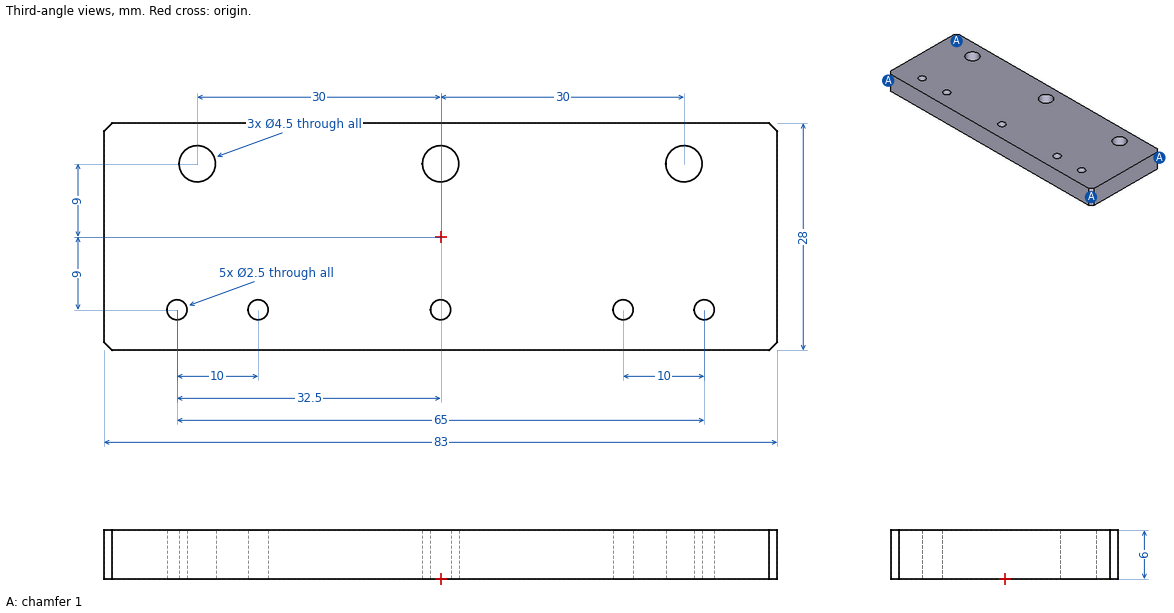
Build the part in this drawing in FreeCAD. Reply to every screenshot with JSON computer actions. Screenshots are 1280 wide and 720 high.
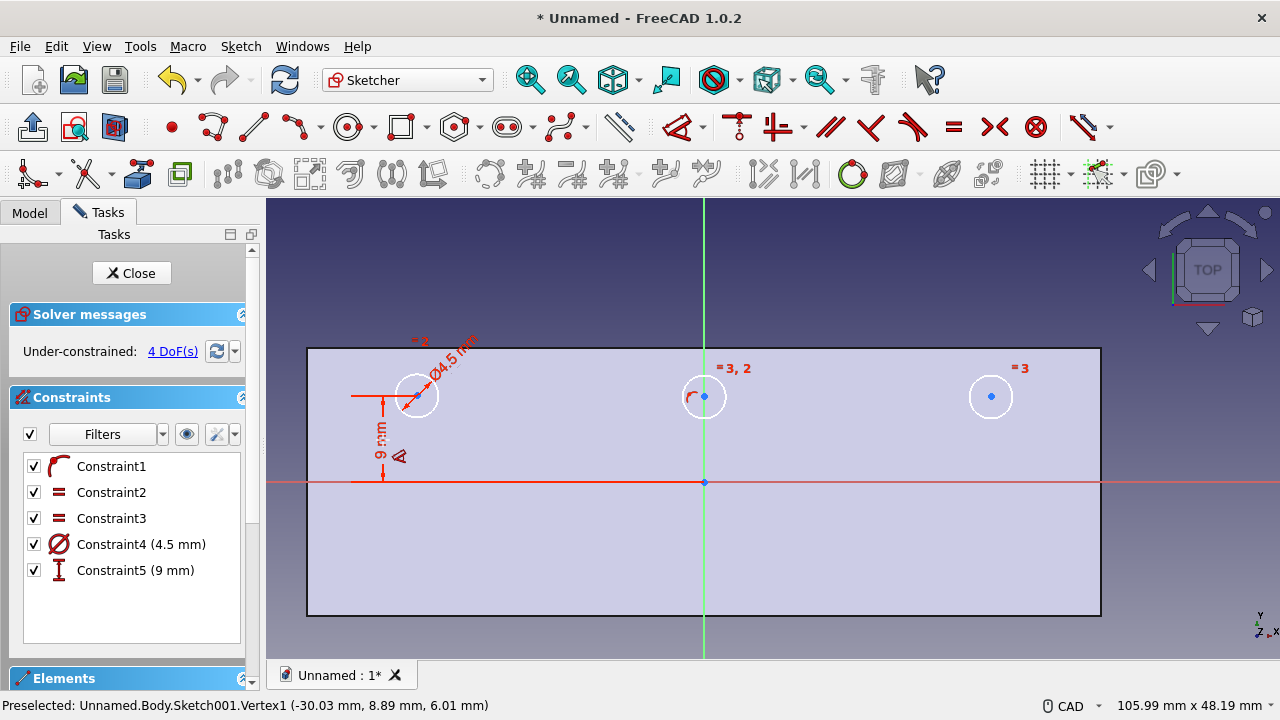
{"action": "left_click", "coordinate": [704, 397]}
{"action": "left_click", "coordinate": [738, 440]}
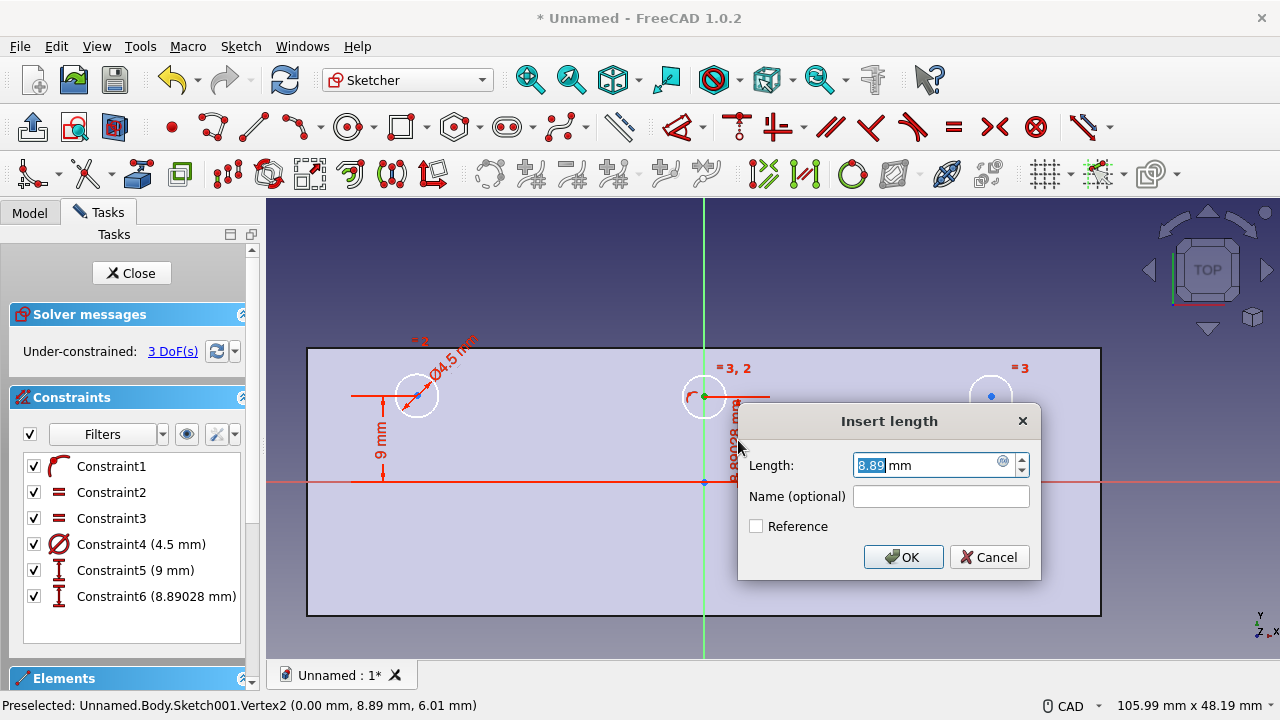
{"action": "type", "text": "9"}
{"action": "key", "text": "Return"}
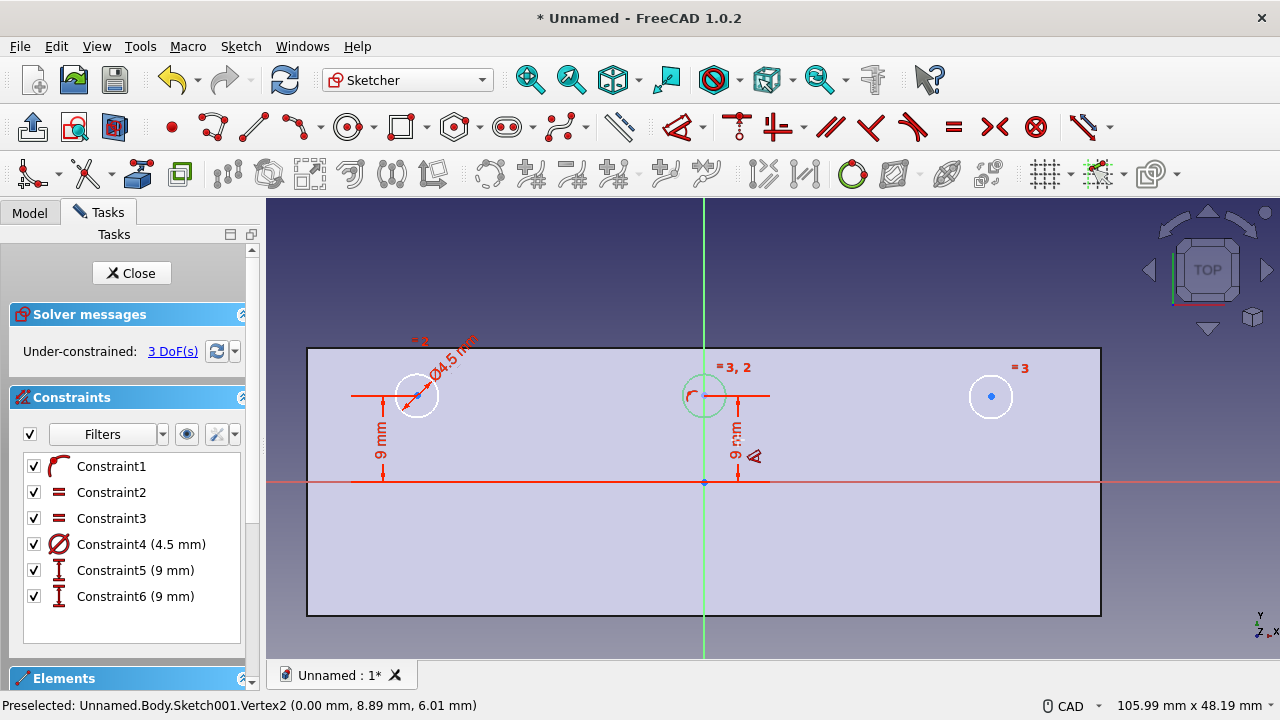
{"action": "left_click", "coordinate": [991, 397]}
{"action": "left_click", "coordinate": [1025, 440]}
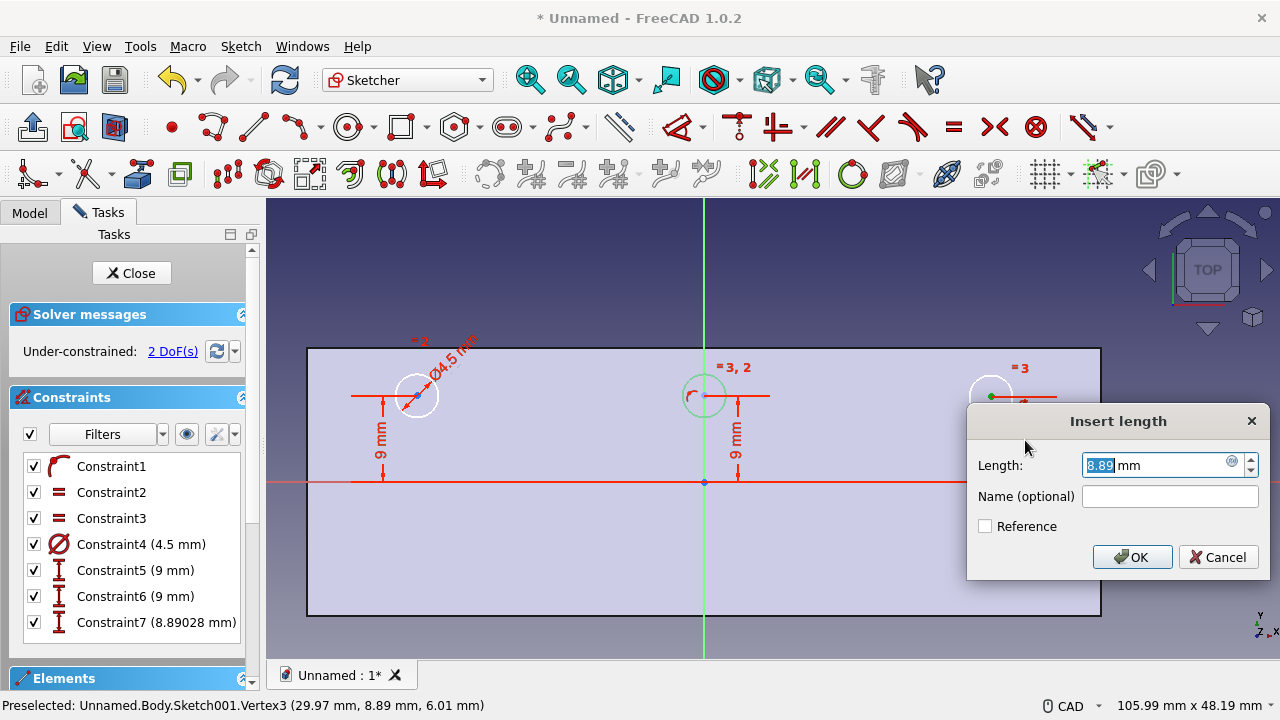
{"action": "type", "text": "9"}
{"action": "key", "text": "Return"}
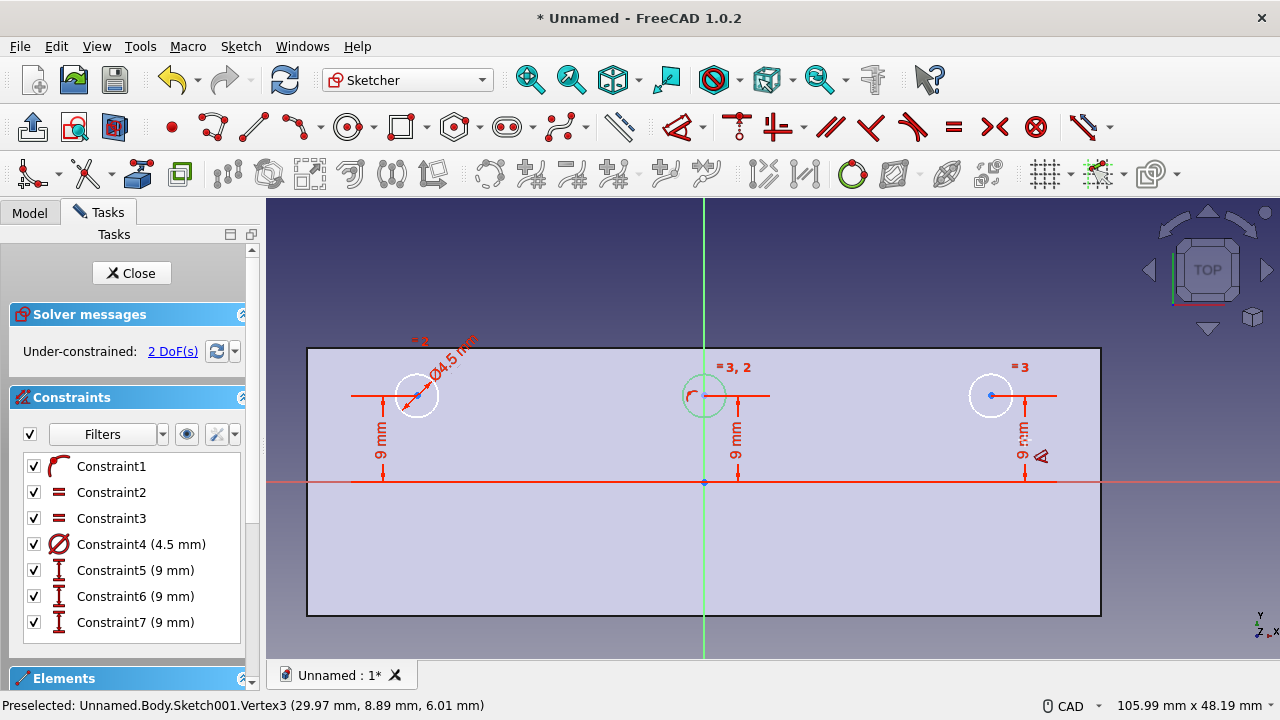
{"action": "left_click", "coordinate": [417, 396]}
{"action": "left_click", "coordinate": [561, 516]}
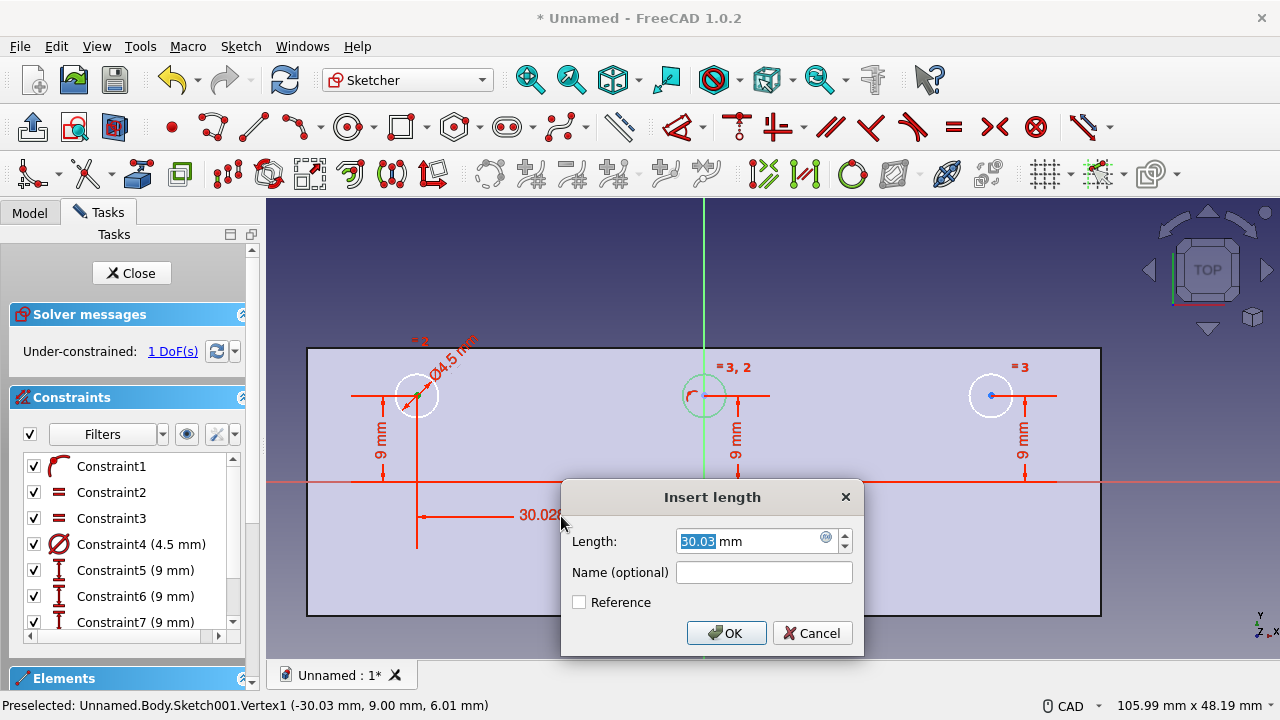
{"action": "type", "text": "30"}
{"action": "key", "text": "Return"}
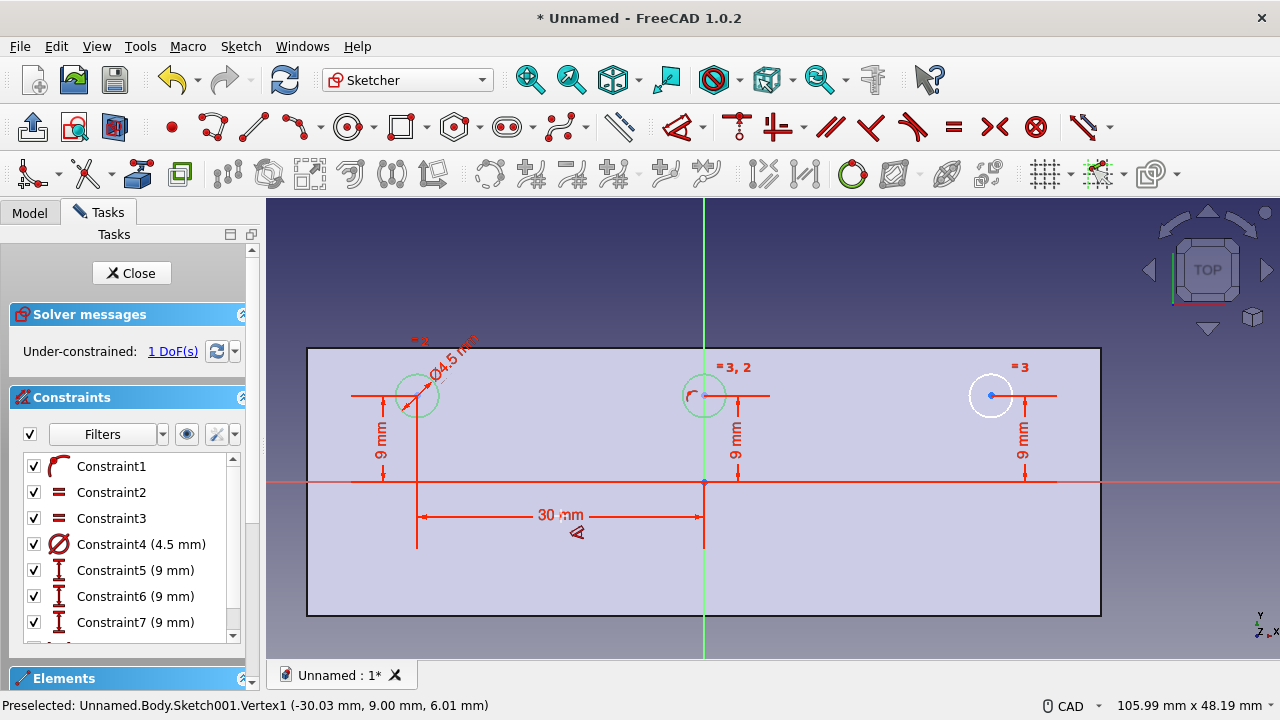
{"action": "left_click", "coordinate": [991, 396]}
{"action": "left_click", "coordinate": [848, 516]}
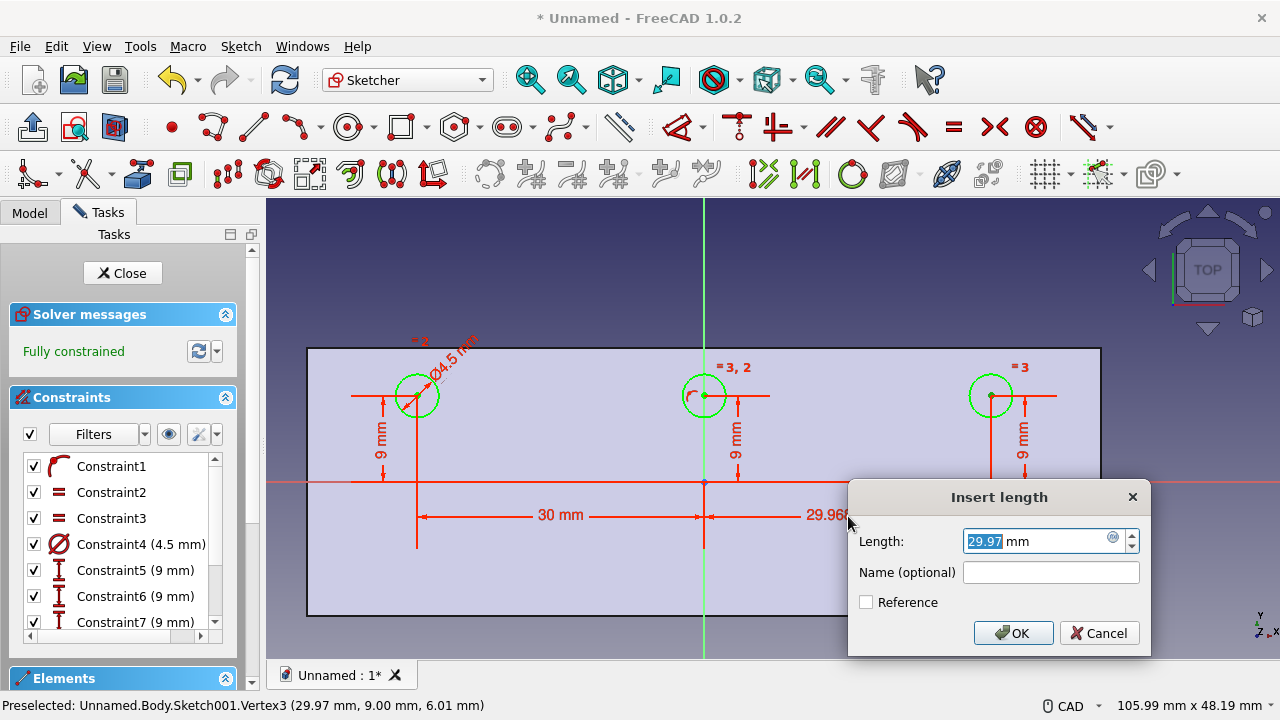
{"action": "type", "text": "30"}
{"action": "key", "text": "Return"}
{"action": "key", "text": "Escape"}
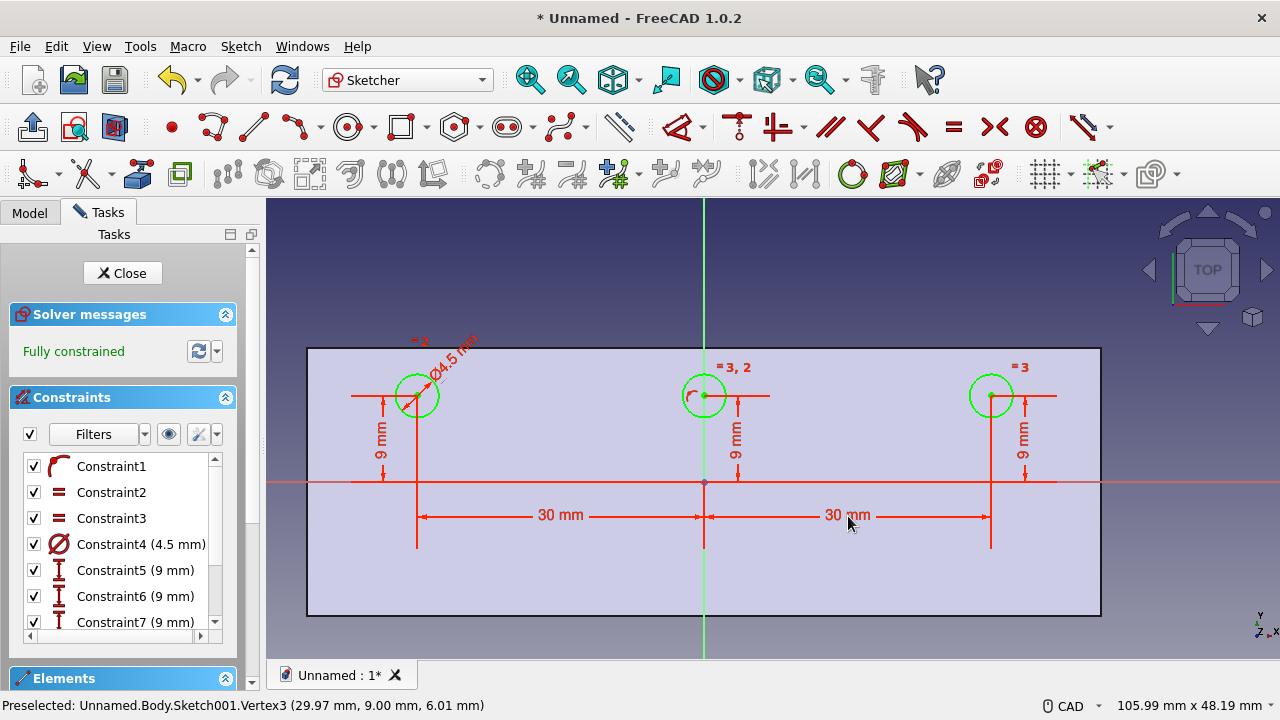
{"action": "left_click", "coordinate": [123, 273]}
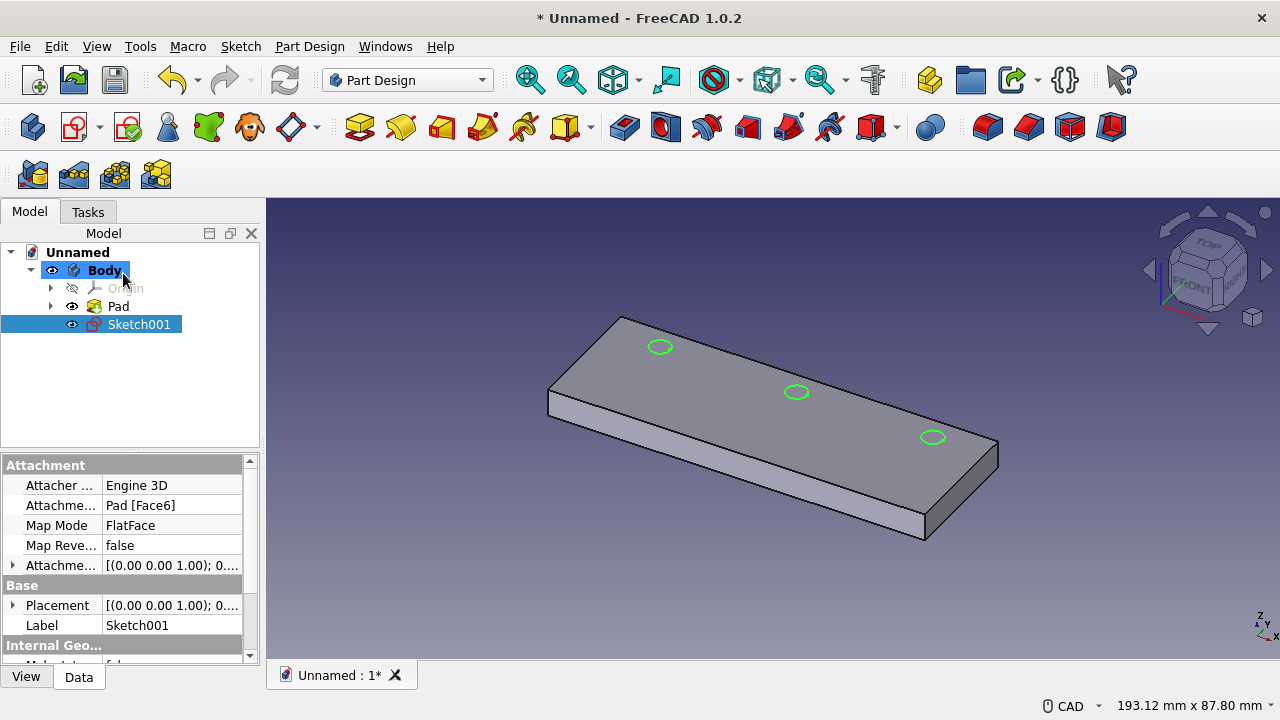
{"action": "left_click", "coordinate": [666, 128]}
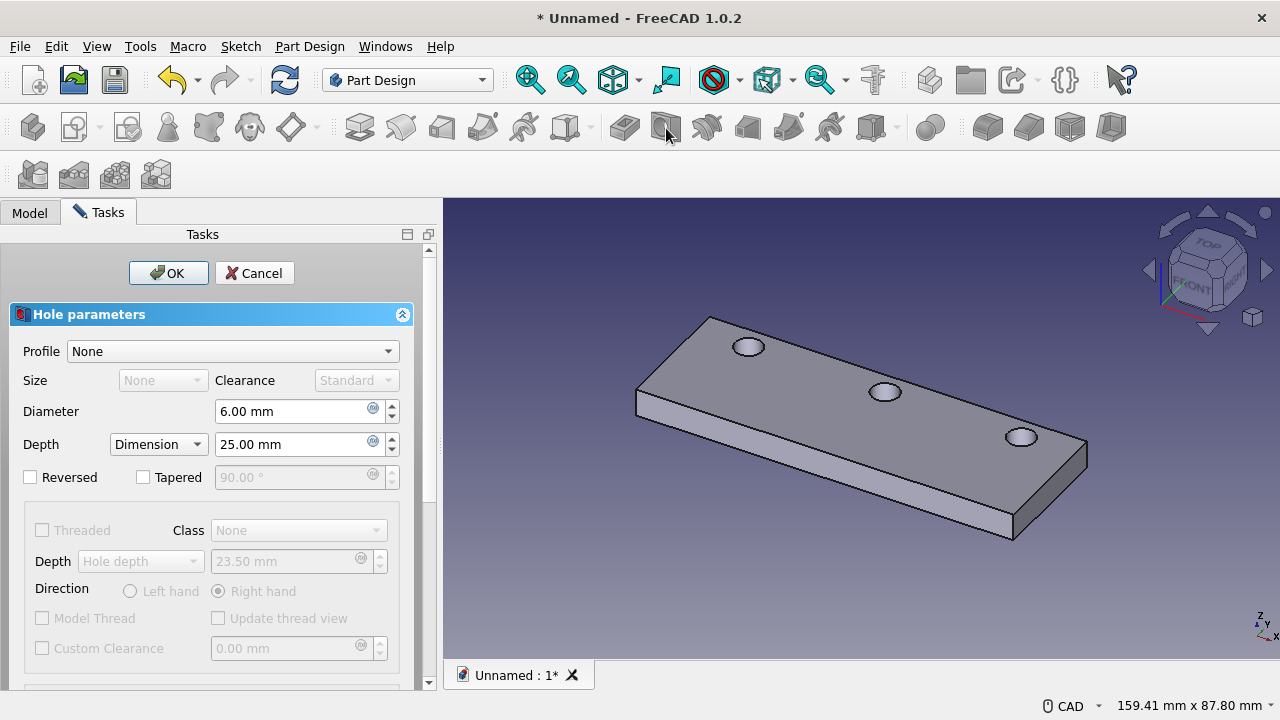
{"action": "triple_click", "coordinate": [300, 412]}